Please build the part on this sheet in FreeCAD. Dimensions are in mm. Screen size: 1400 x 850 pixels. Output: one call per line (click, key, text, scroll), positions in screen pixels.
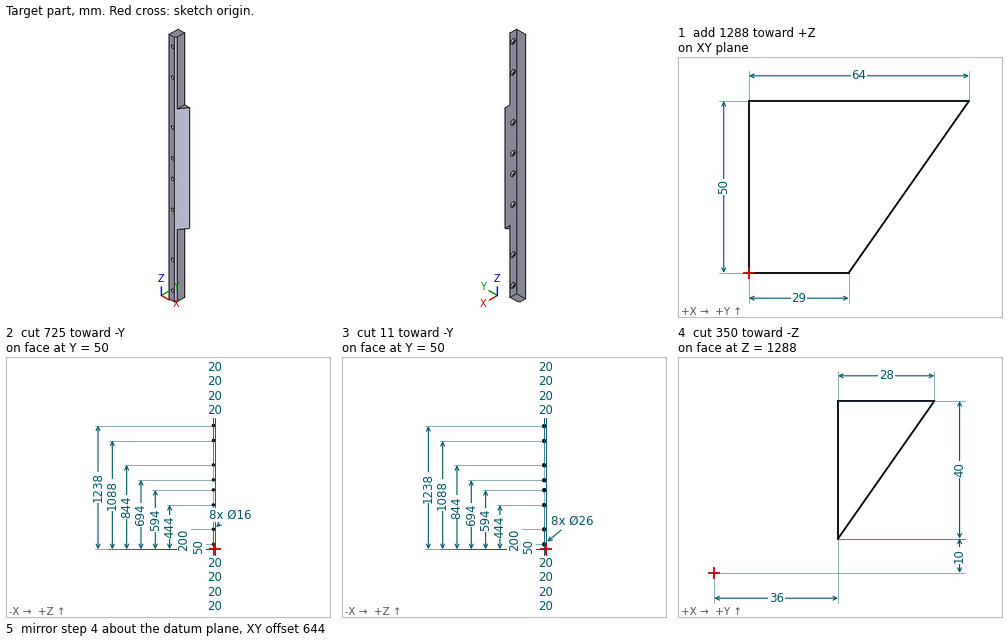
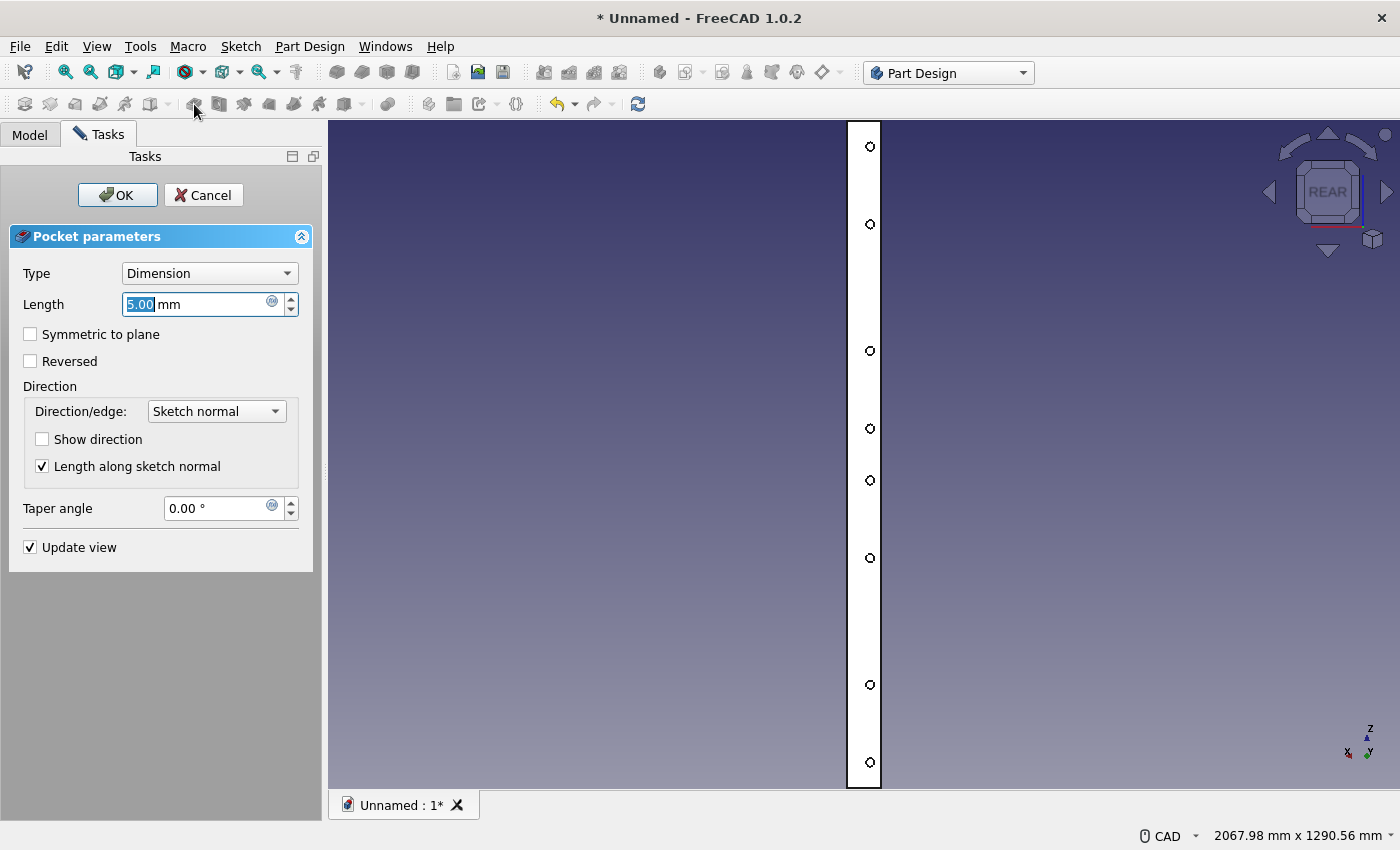
text(725)
key(Tab)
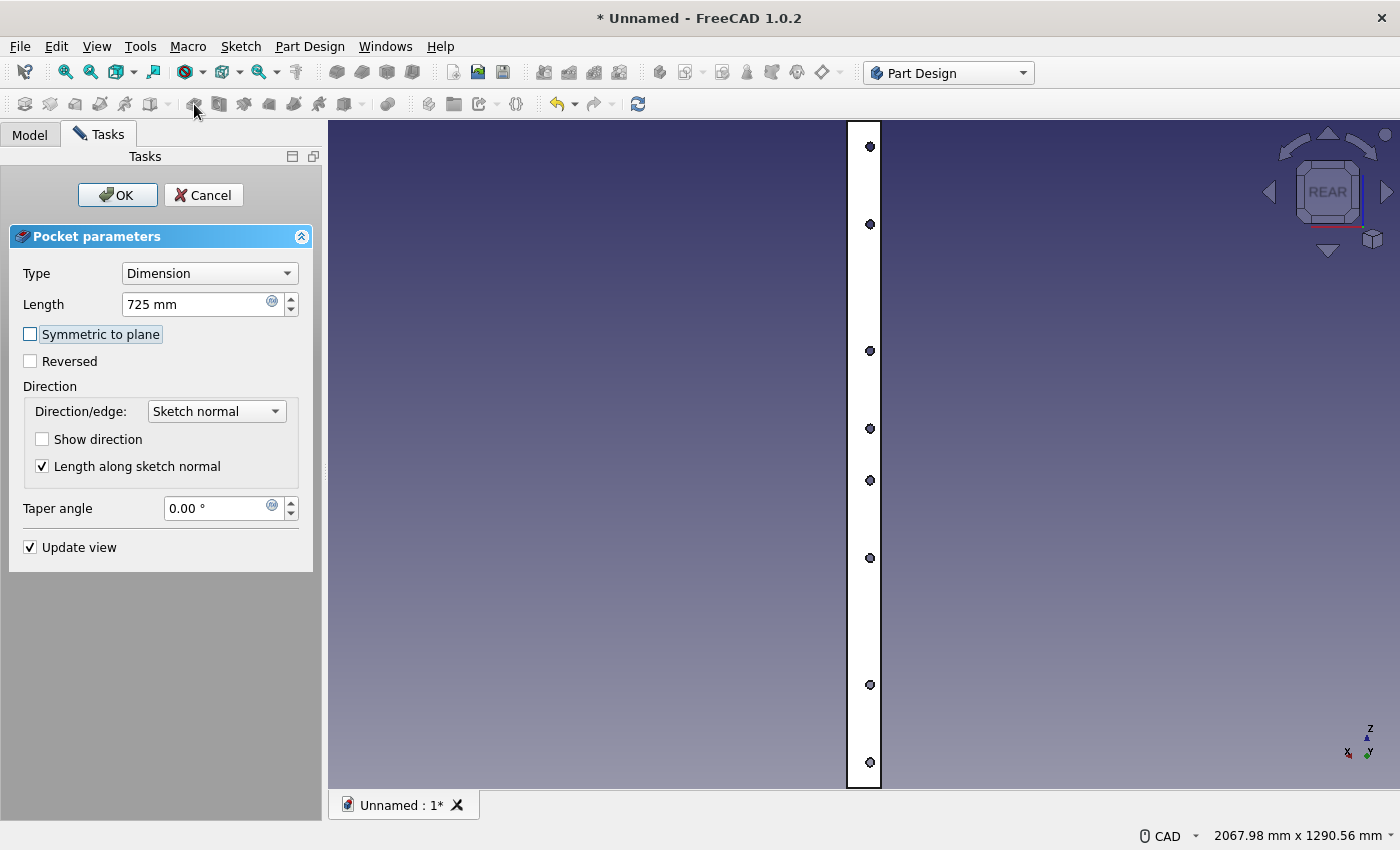
click(118, 195)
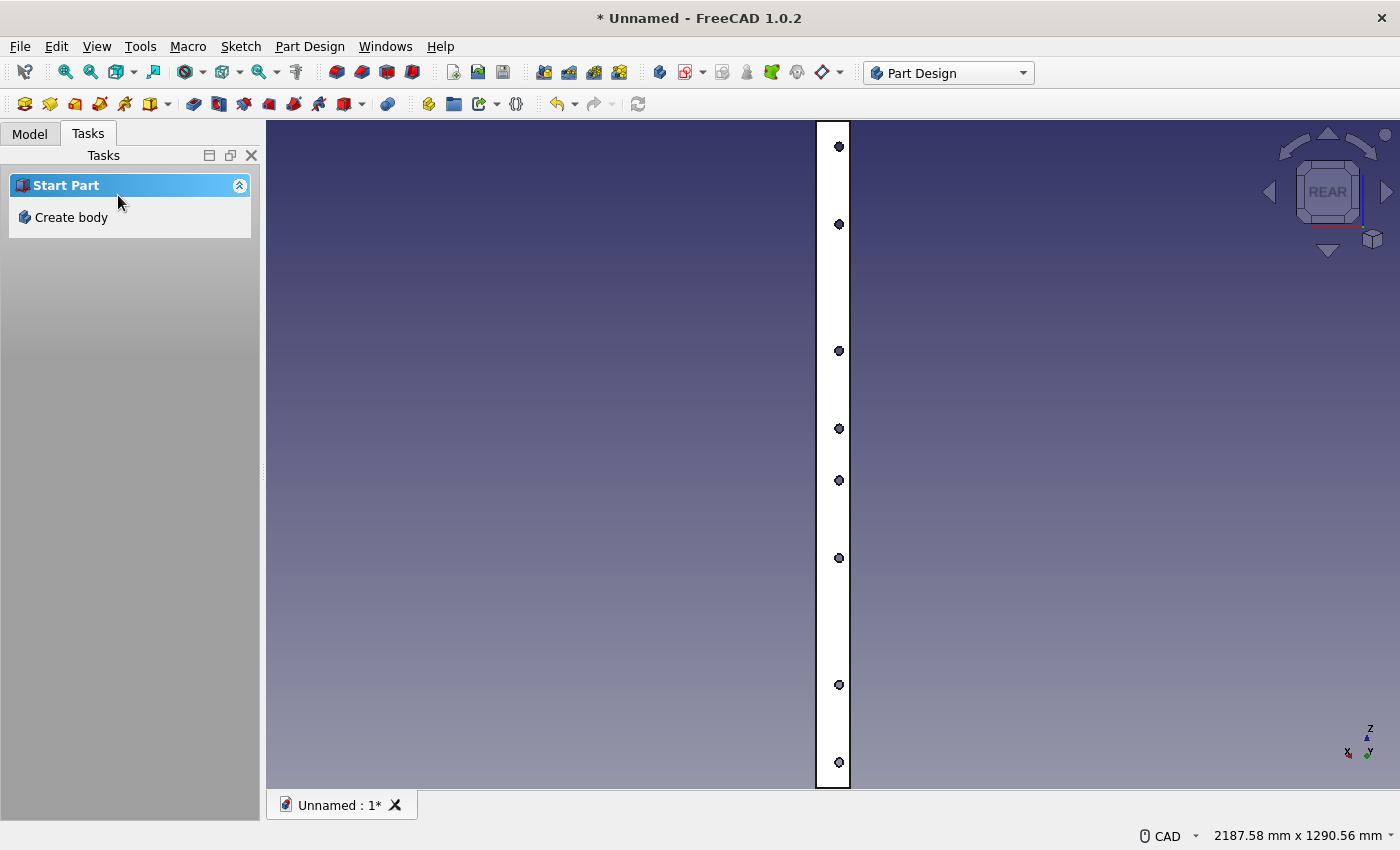
click(833, 167)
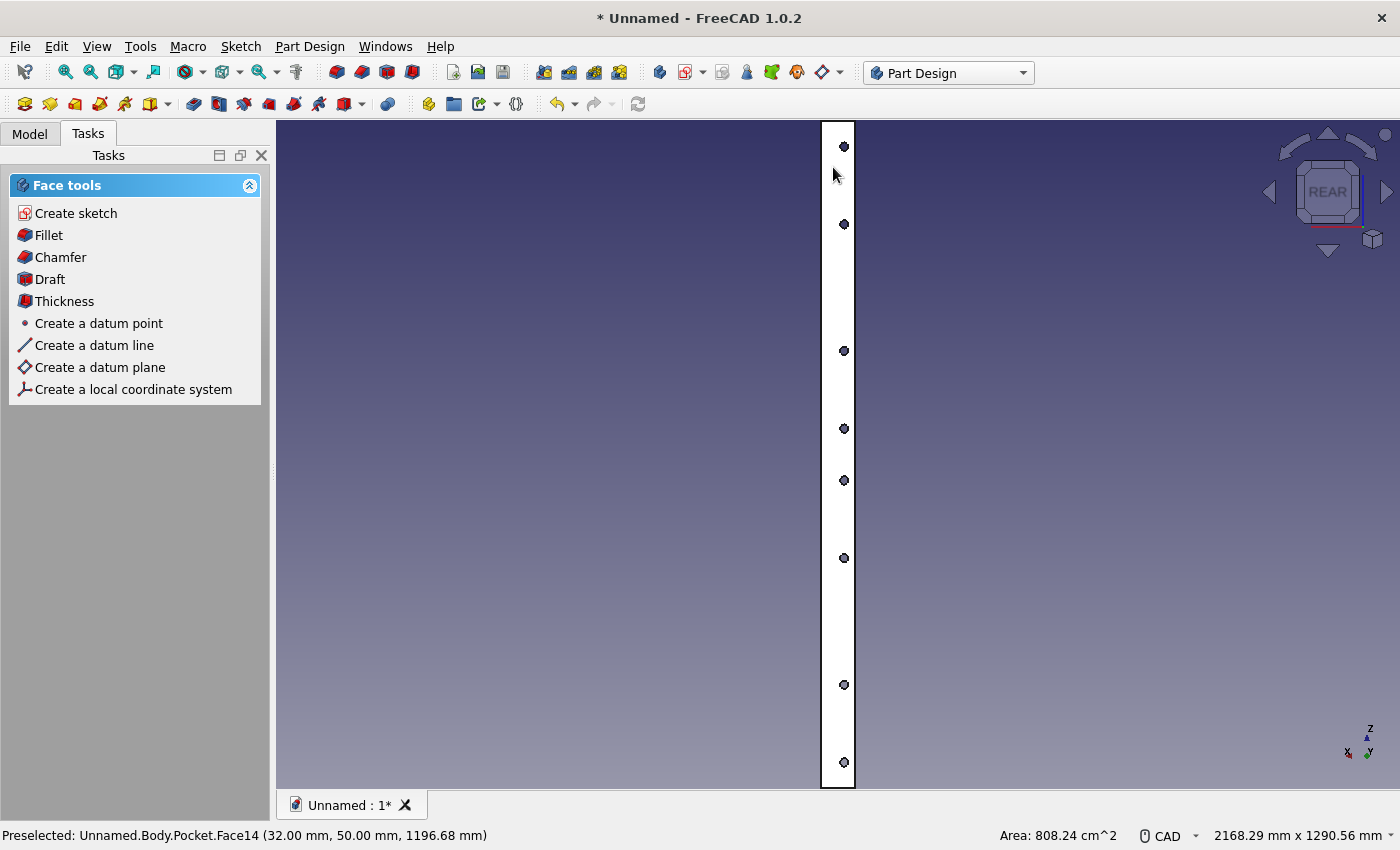
click(684, 72)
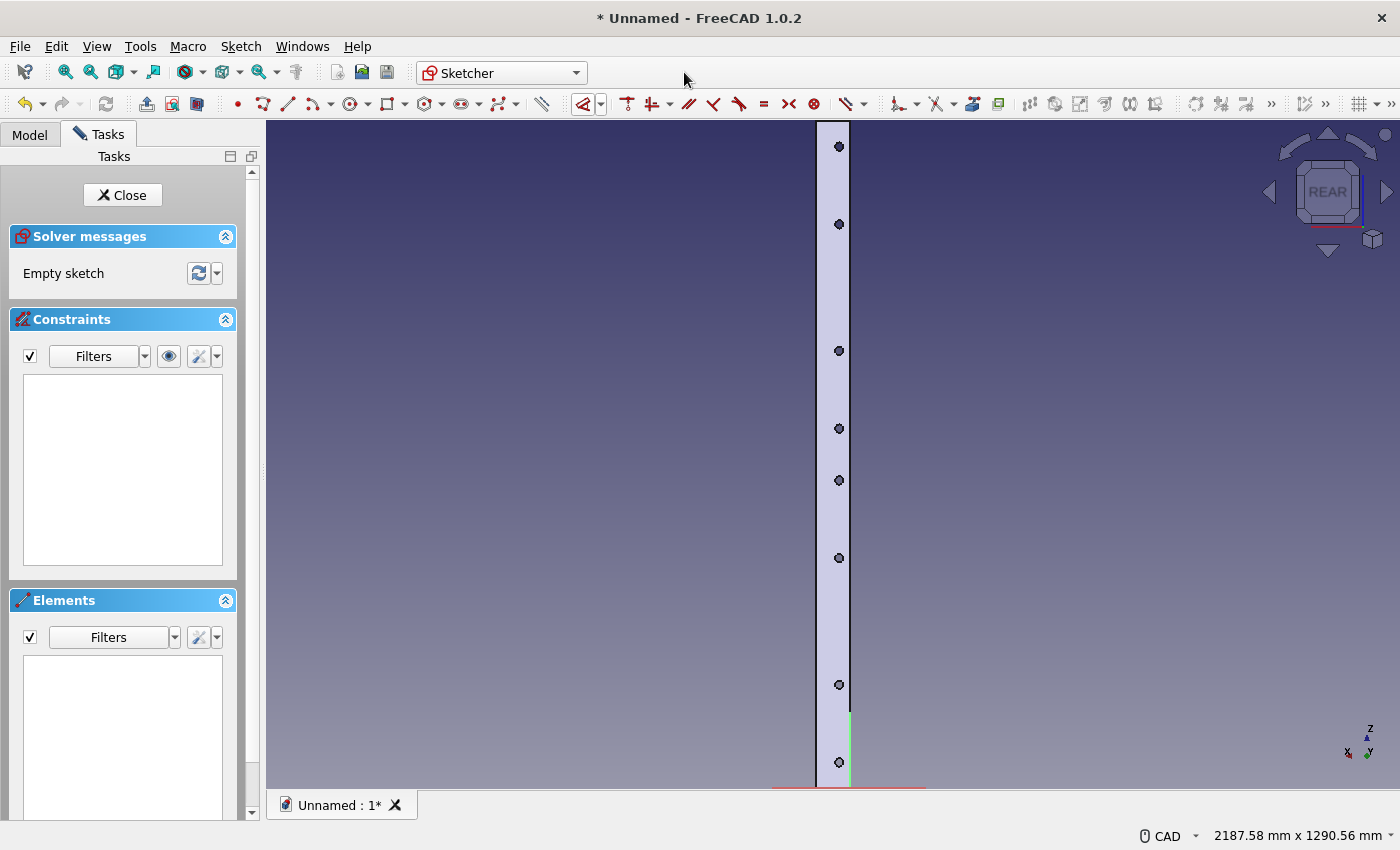
scroll(609, 435, down, 2)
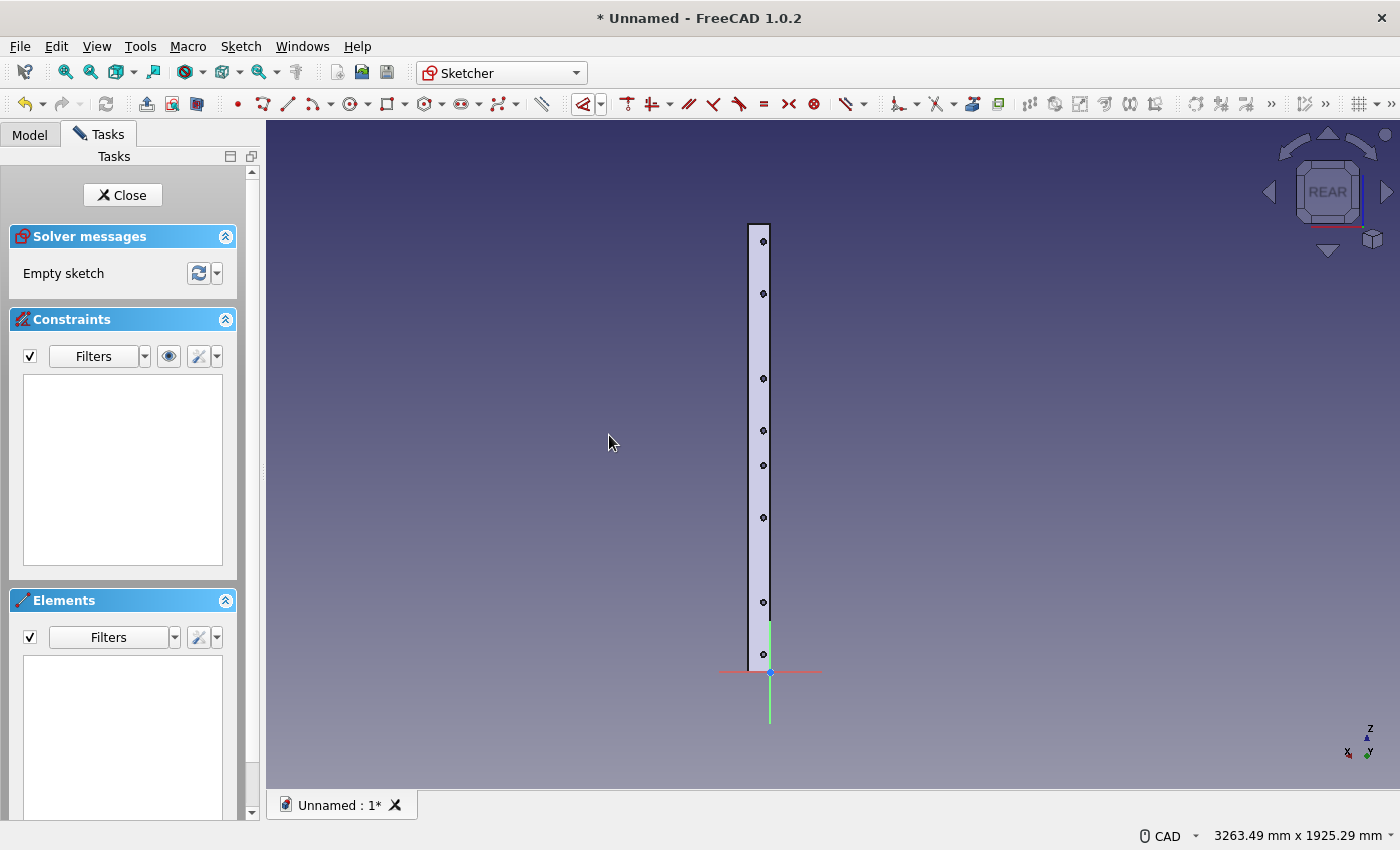
key(g)
key(c)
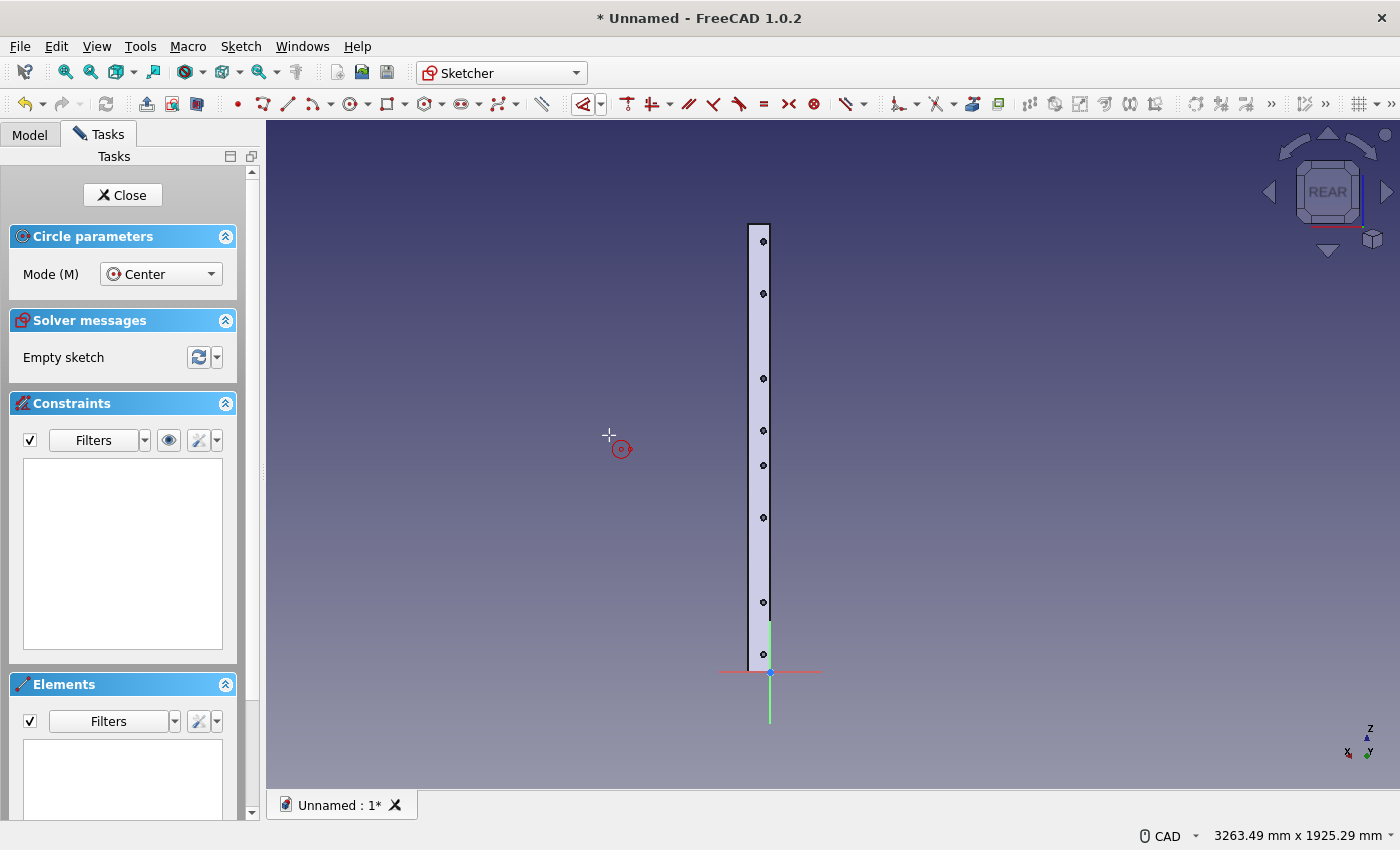
scroll(763, 655, up, 9)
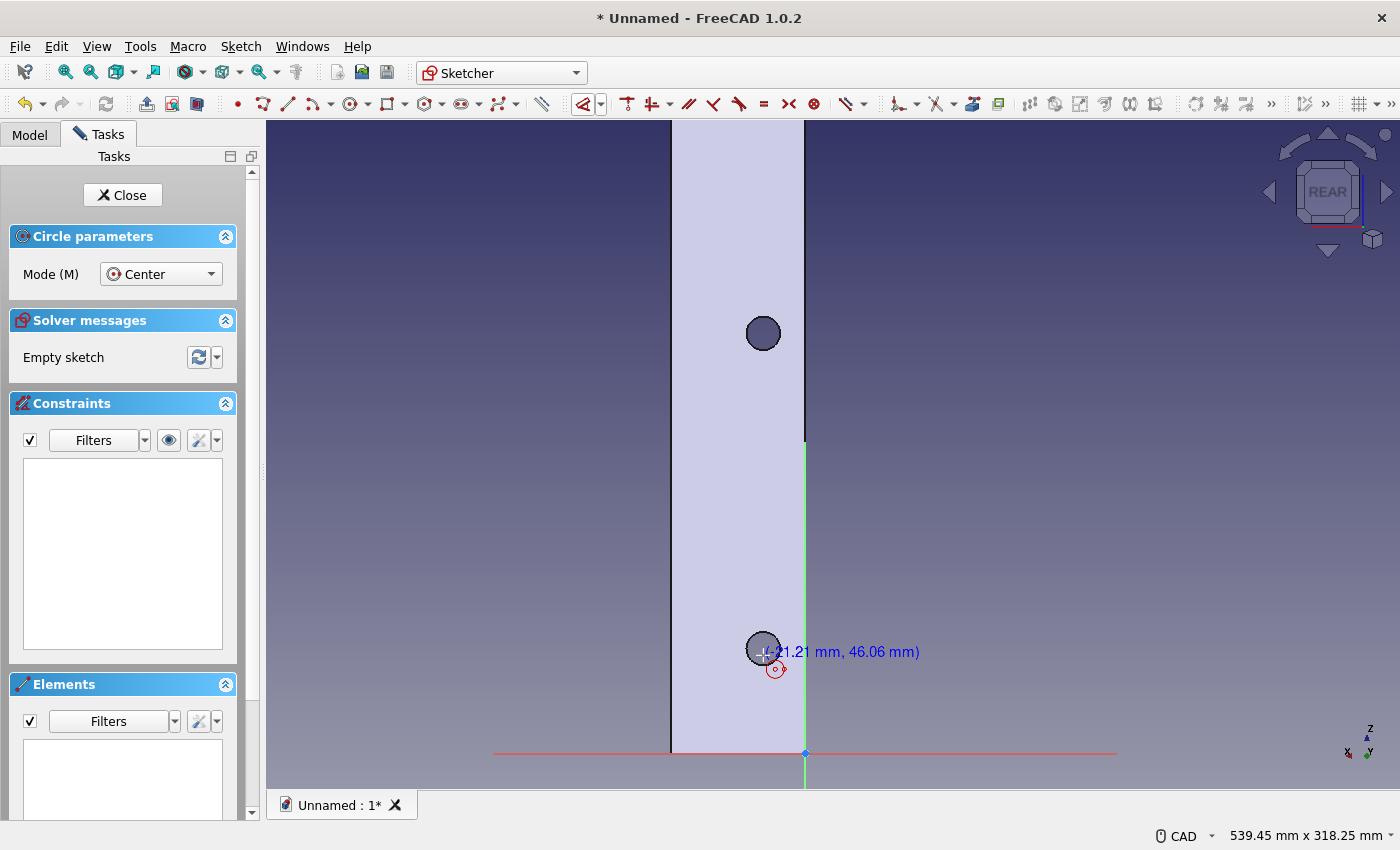
click(763, 649)
click(783, 629)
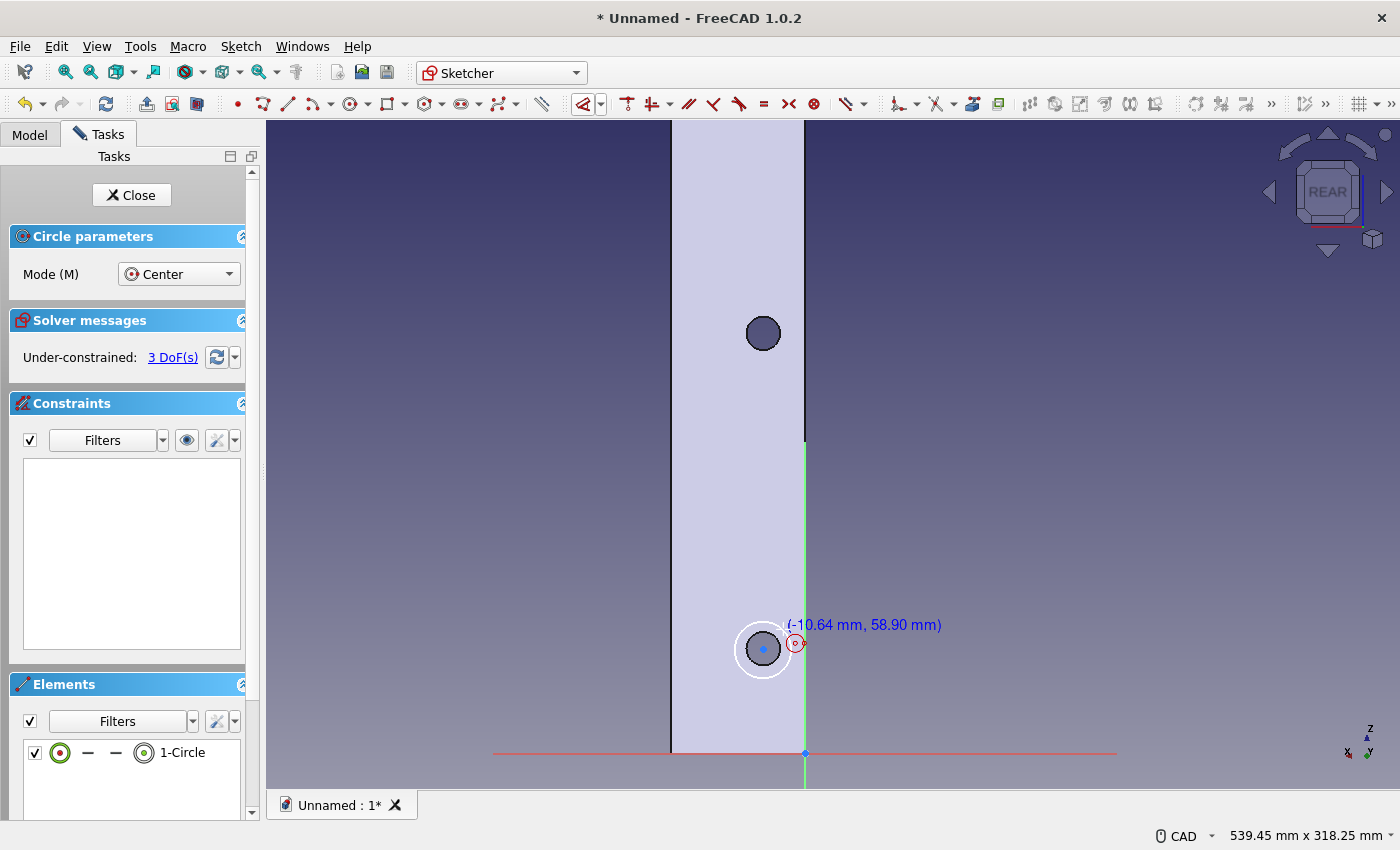
click(763, 333)
click(783, 314)